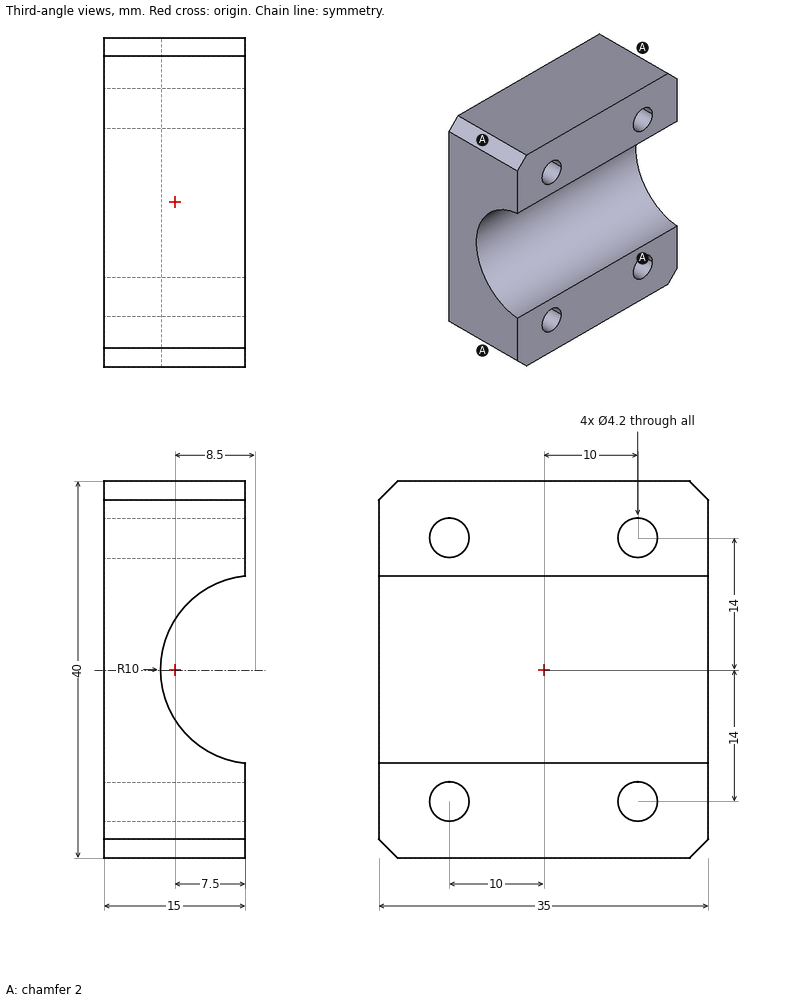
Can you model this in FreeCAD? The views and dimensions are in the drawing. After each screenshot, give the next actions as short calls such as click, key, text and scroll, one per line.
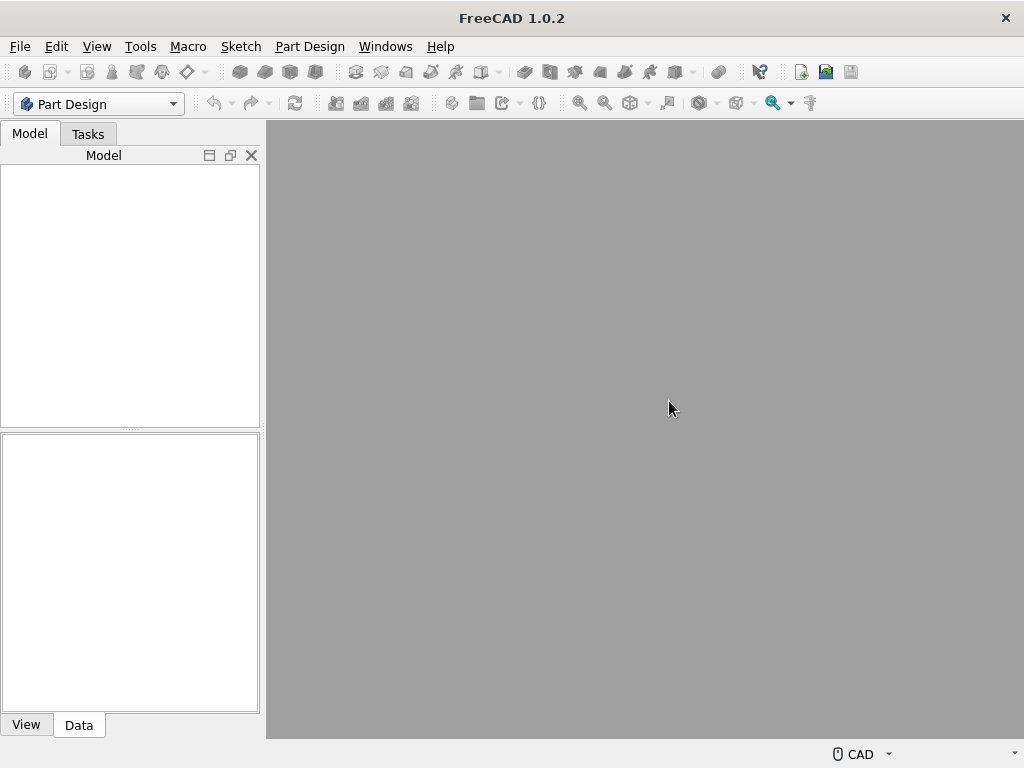
click(801, 72)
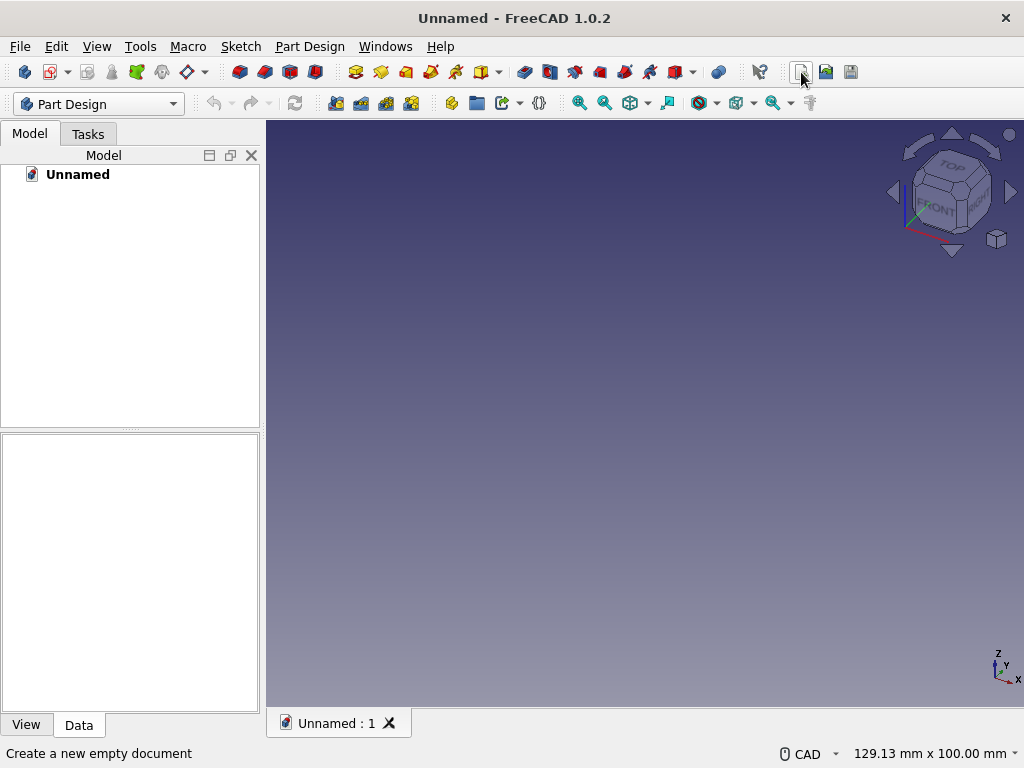
click(50, 72)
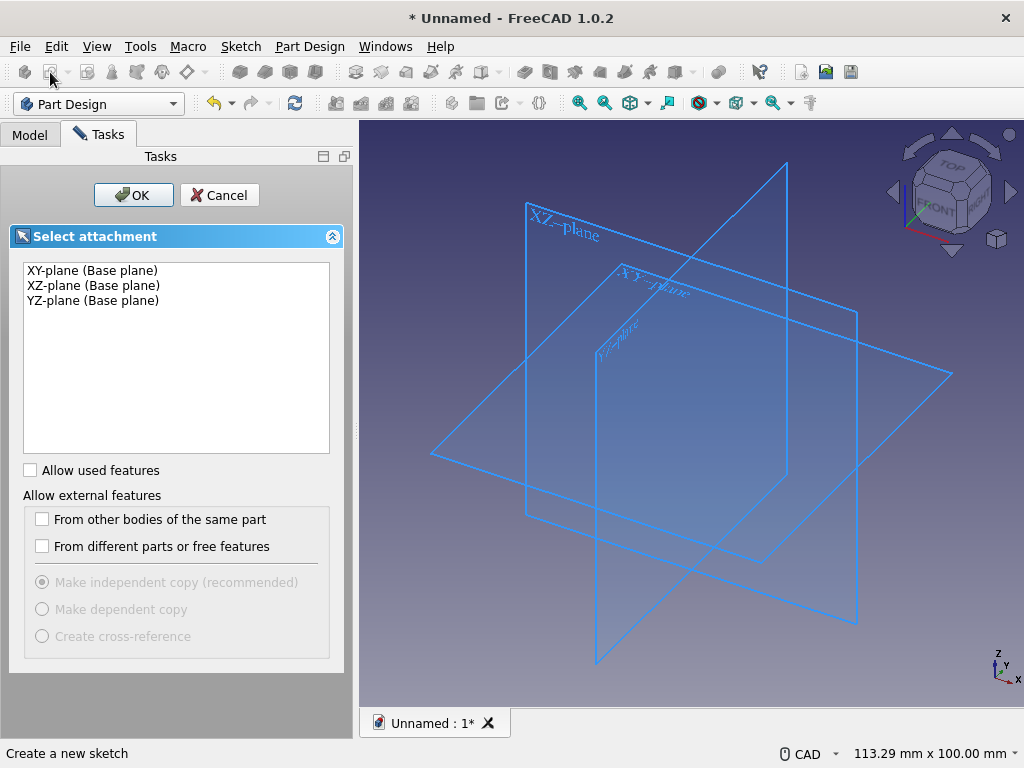
click(84, 286)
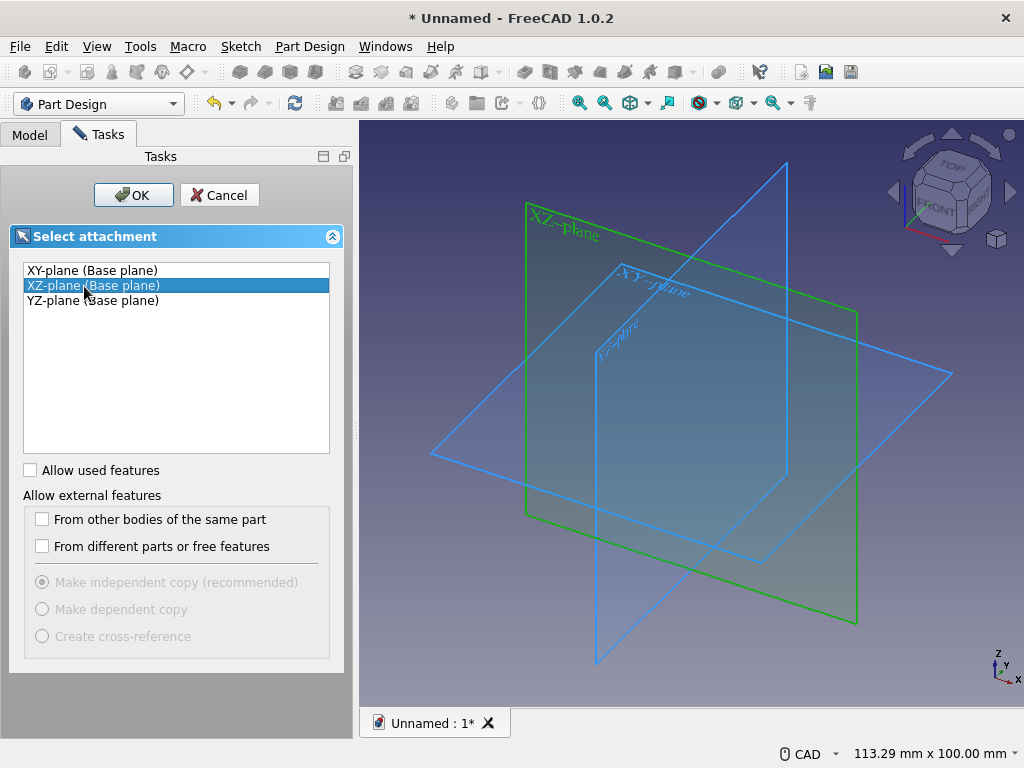
click(134, 195)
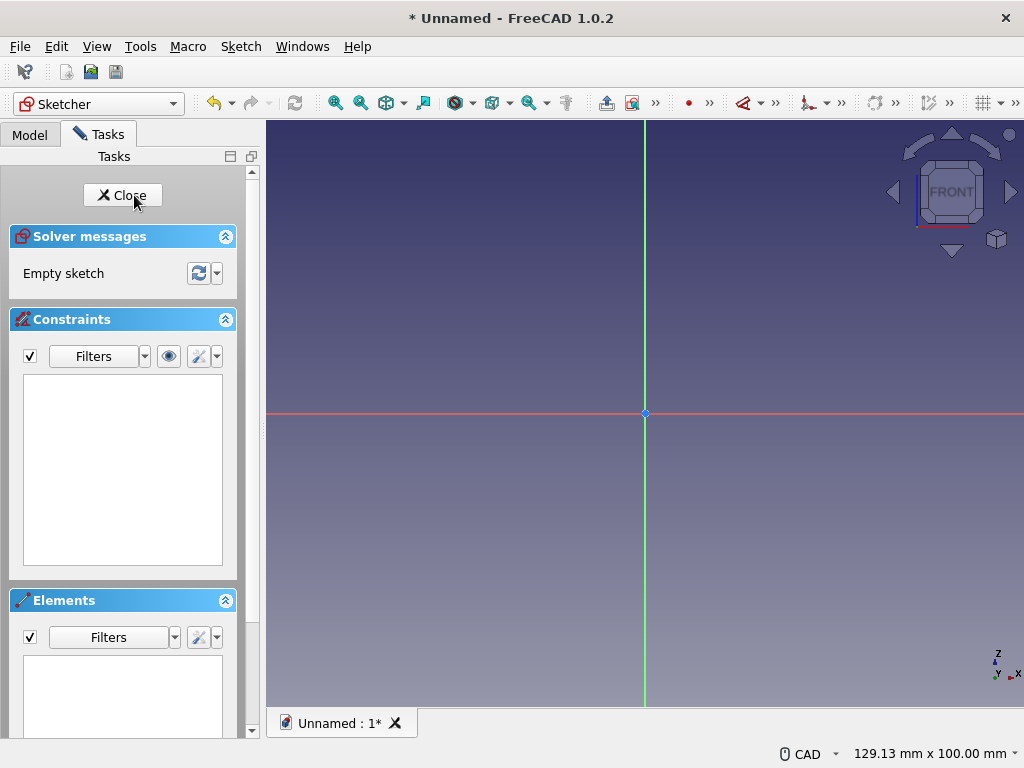
scroll(784, 413, up, 2)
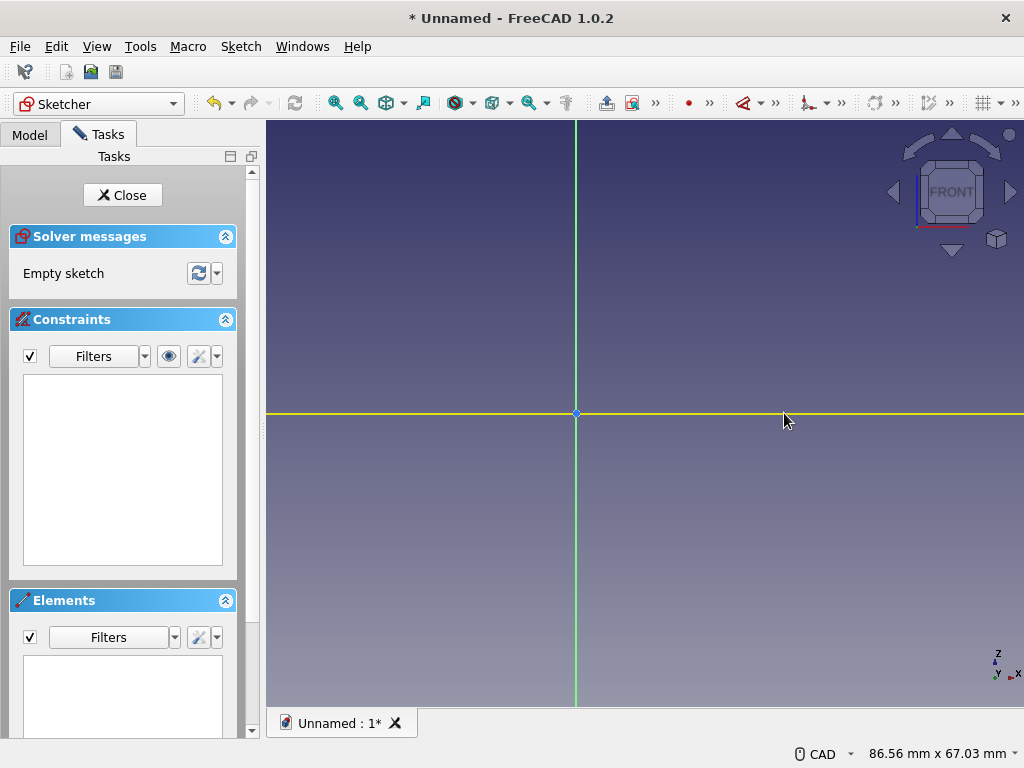
key(g)
key(m)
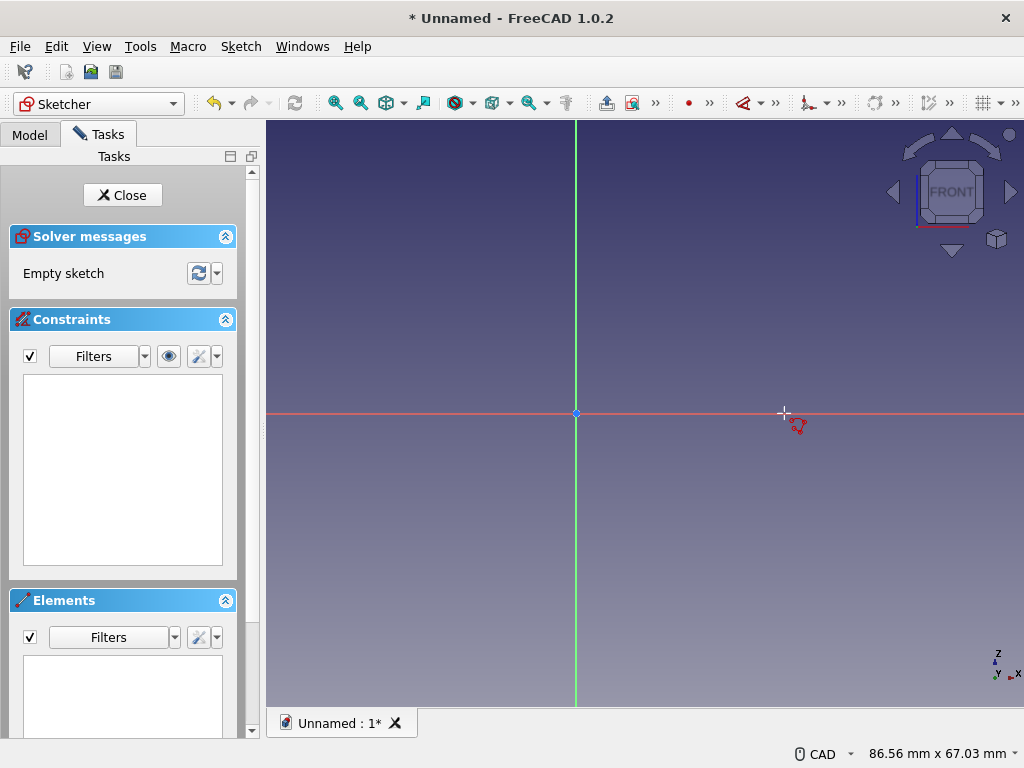
click(642, 501)
click(642, 589)
click(511, 589)
click(511, 238)
click(642, 238)
click(642, 326)
right_click(642, 326)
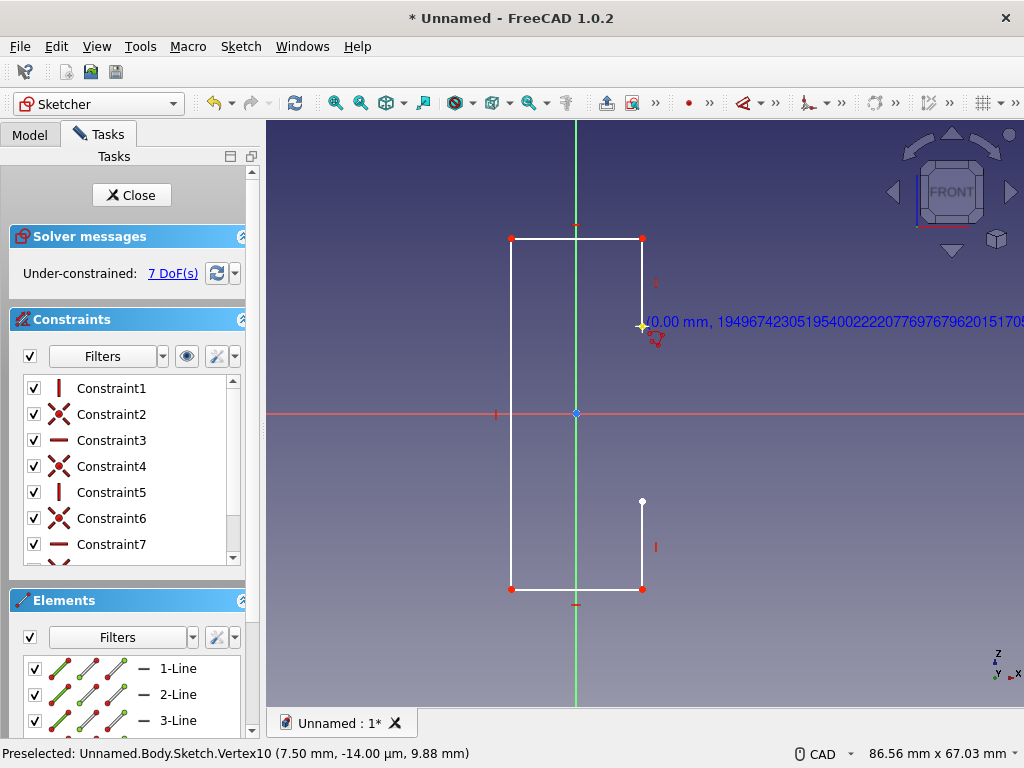
key(g)
key(3)
key(a)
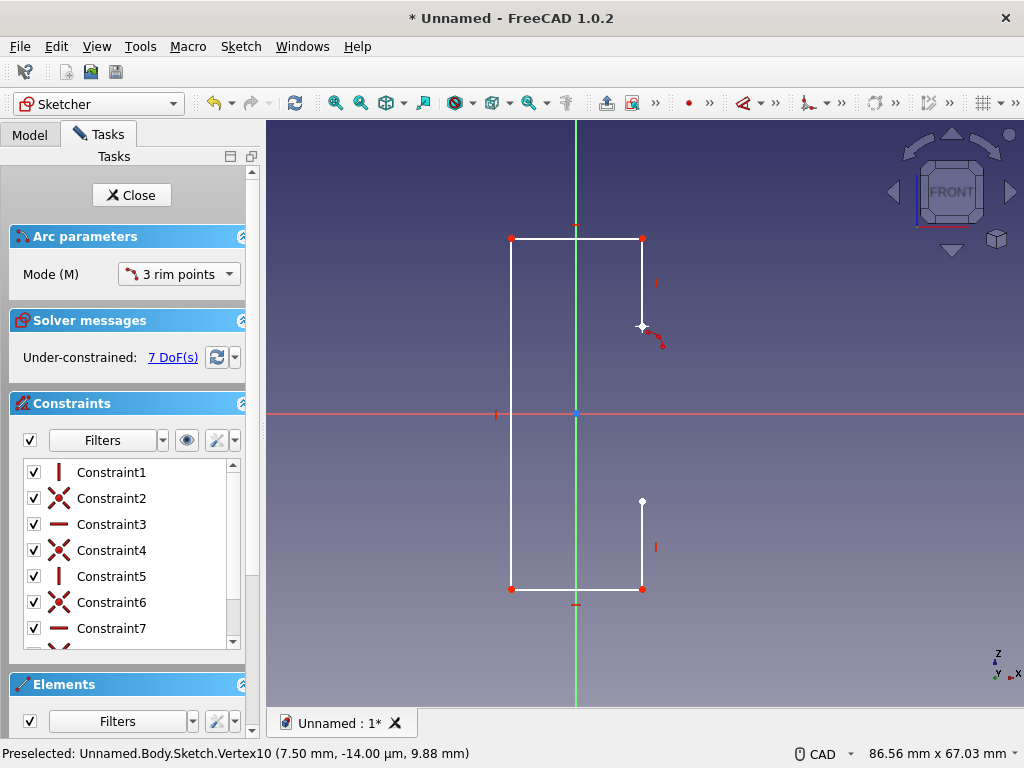
click(642, 327)
click(642, 502)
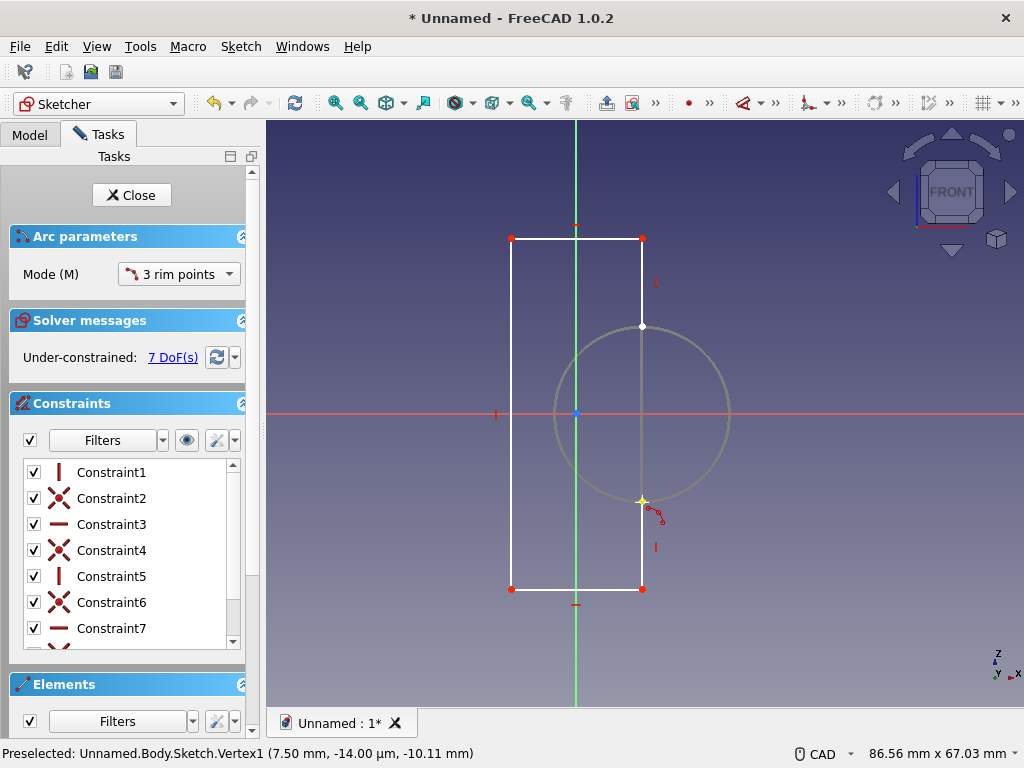
scroll(567, 388, up, 3)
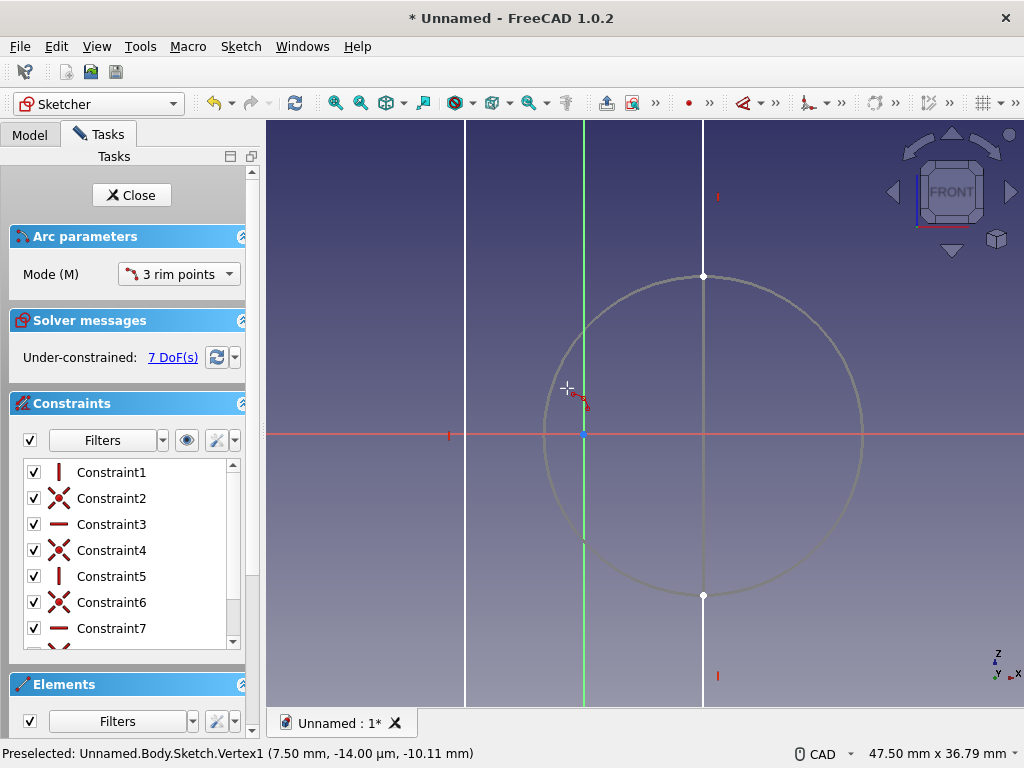
click(567, 388)
key(Escape)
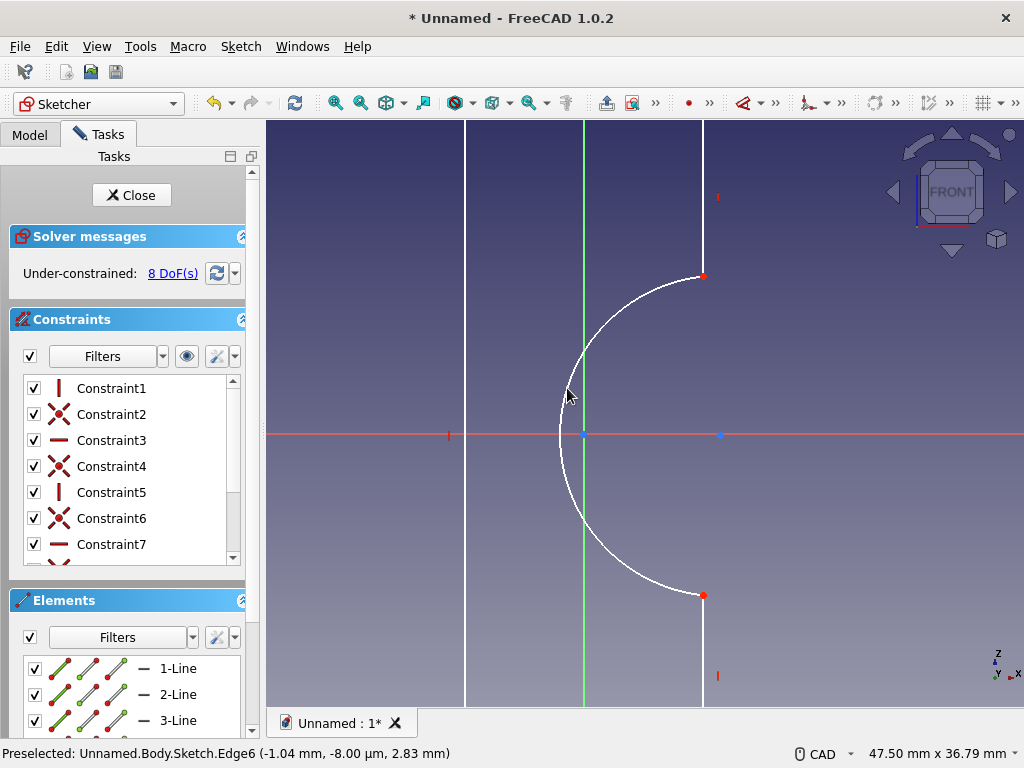
click(720, 436)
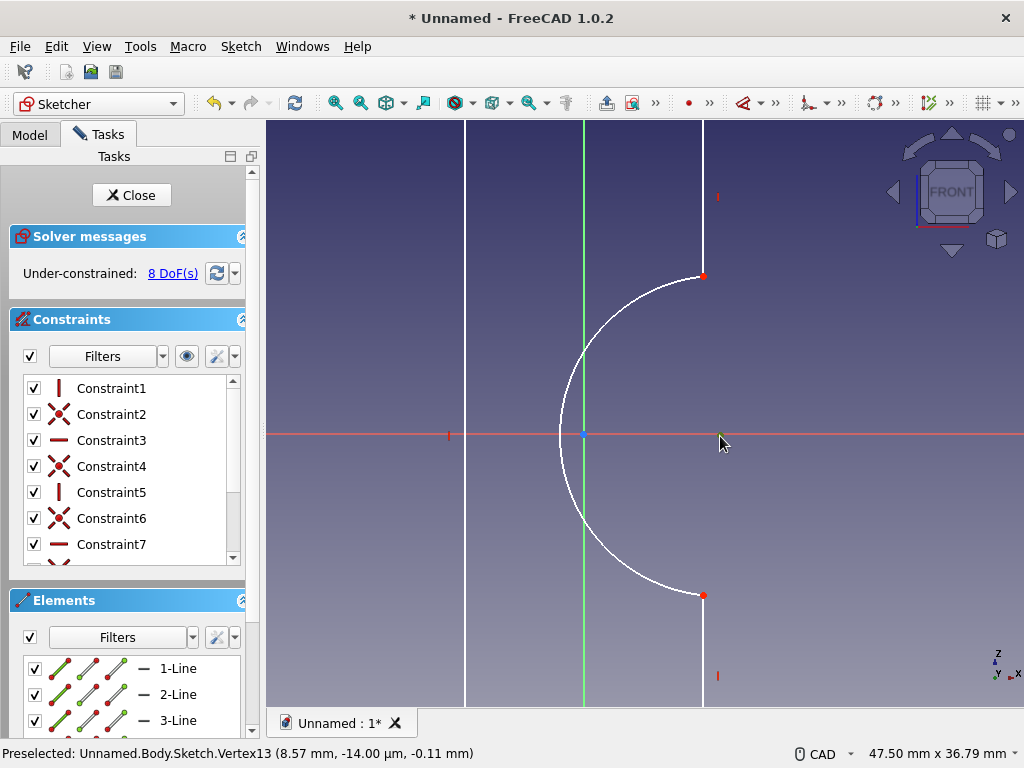
click(334, 434)